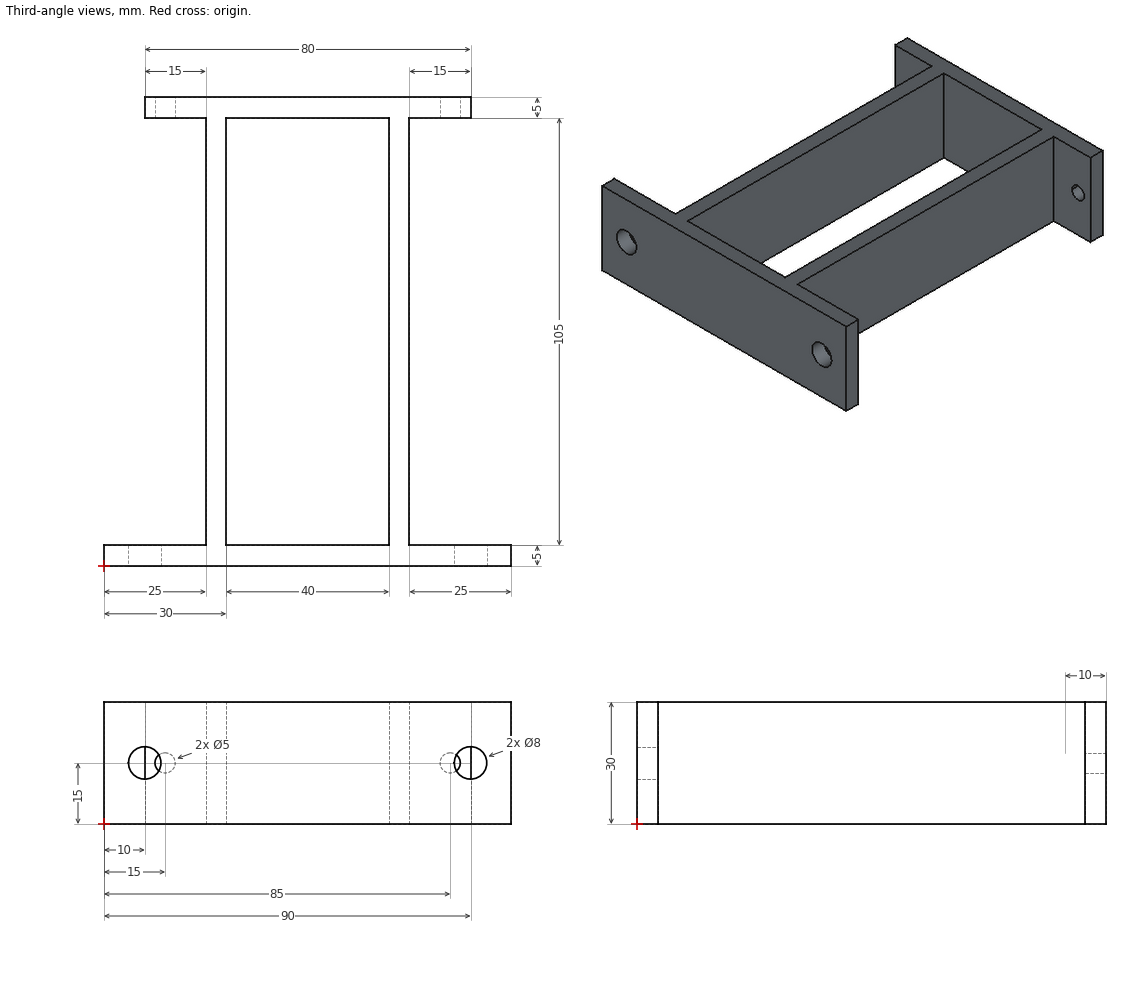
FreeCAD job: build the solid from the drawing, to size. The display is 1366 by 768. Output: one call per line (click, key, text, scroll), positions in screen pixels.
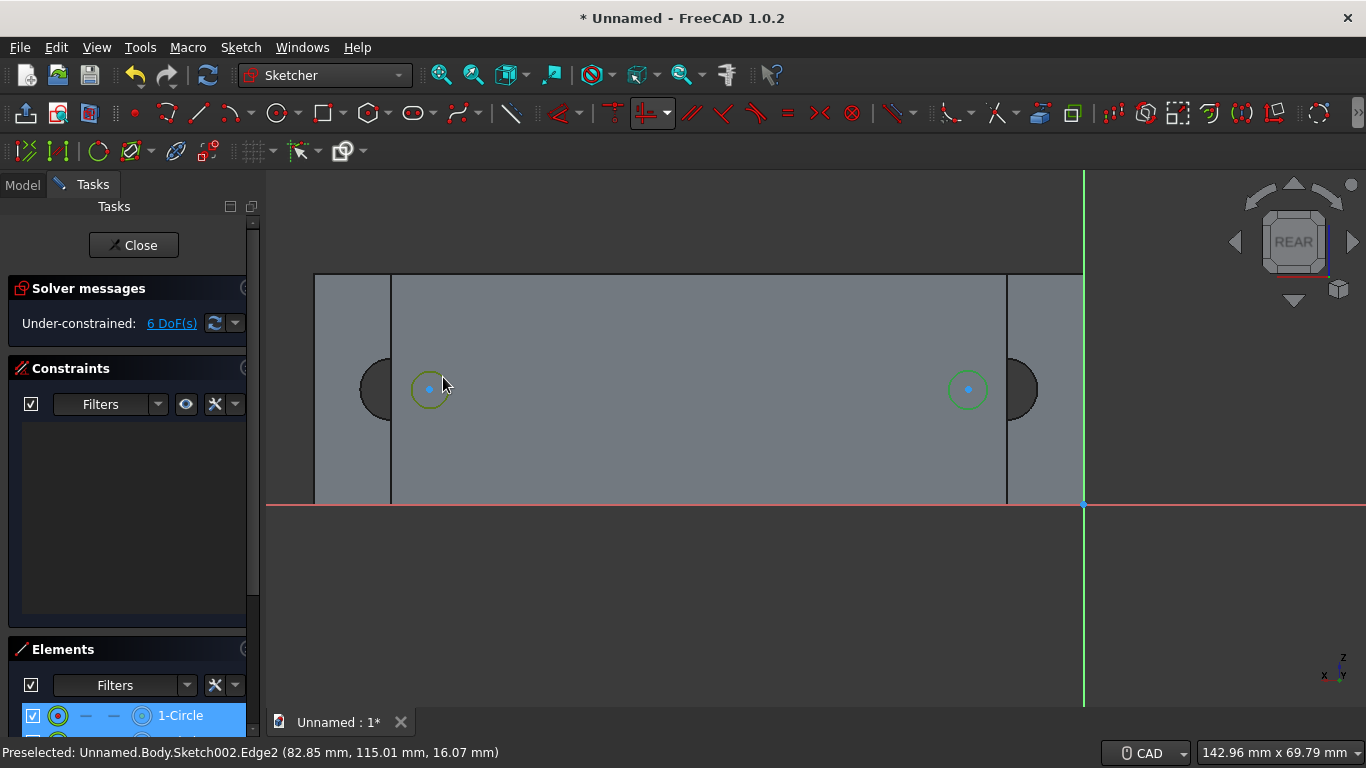
click(788, 114)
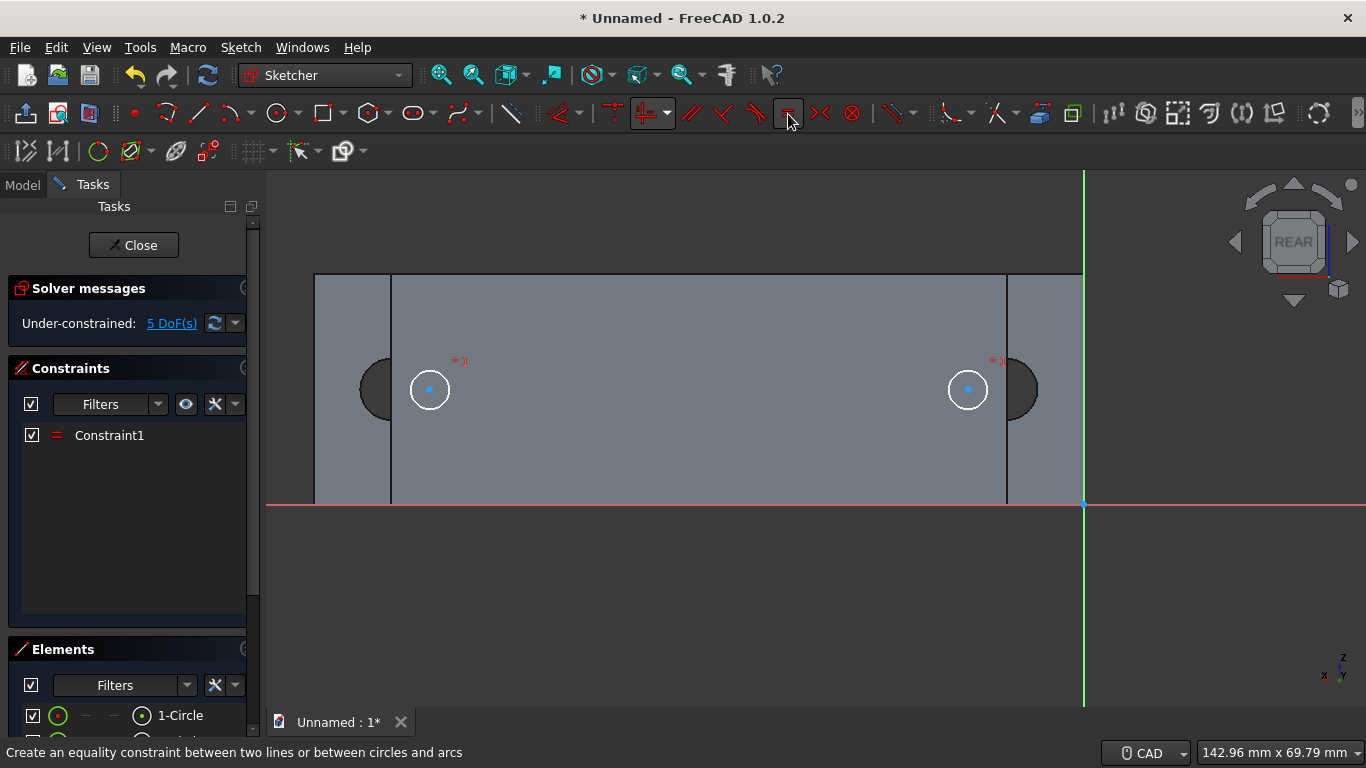
click(968, 390)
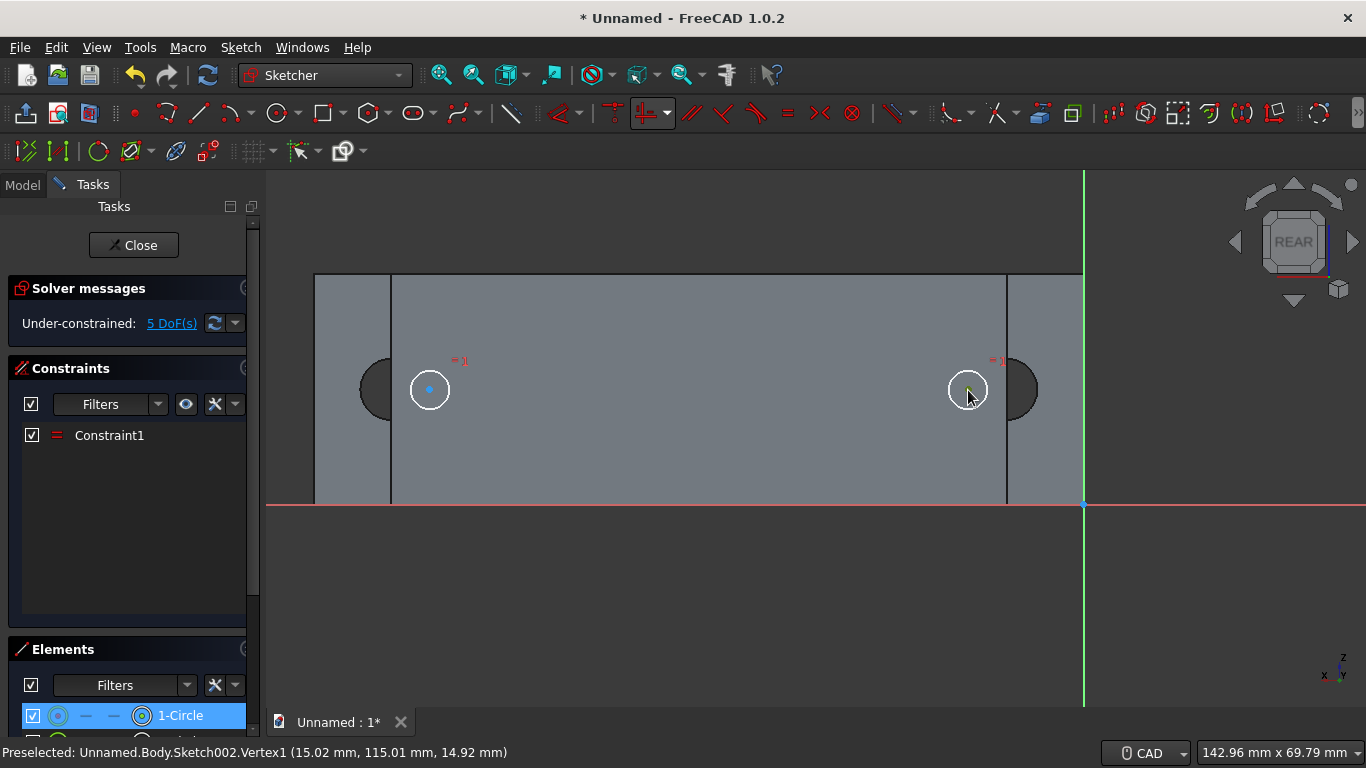
click(430, 390)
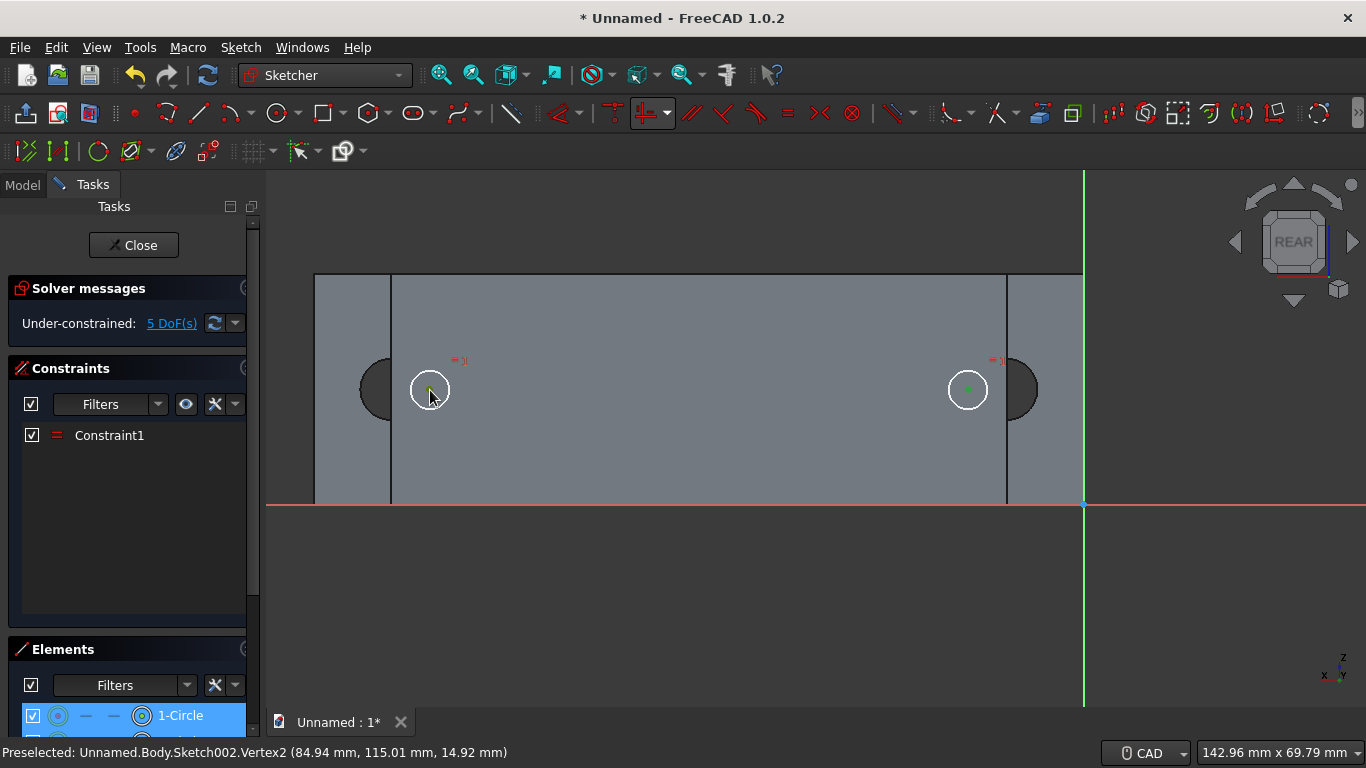
click(670, 114)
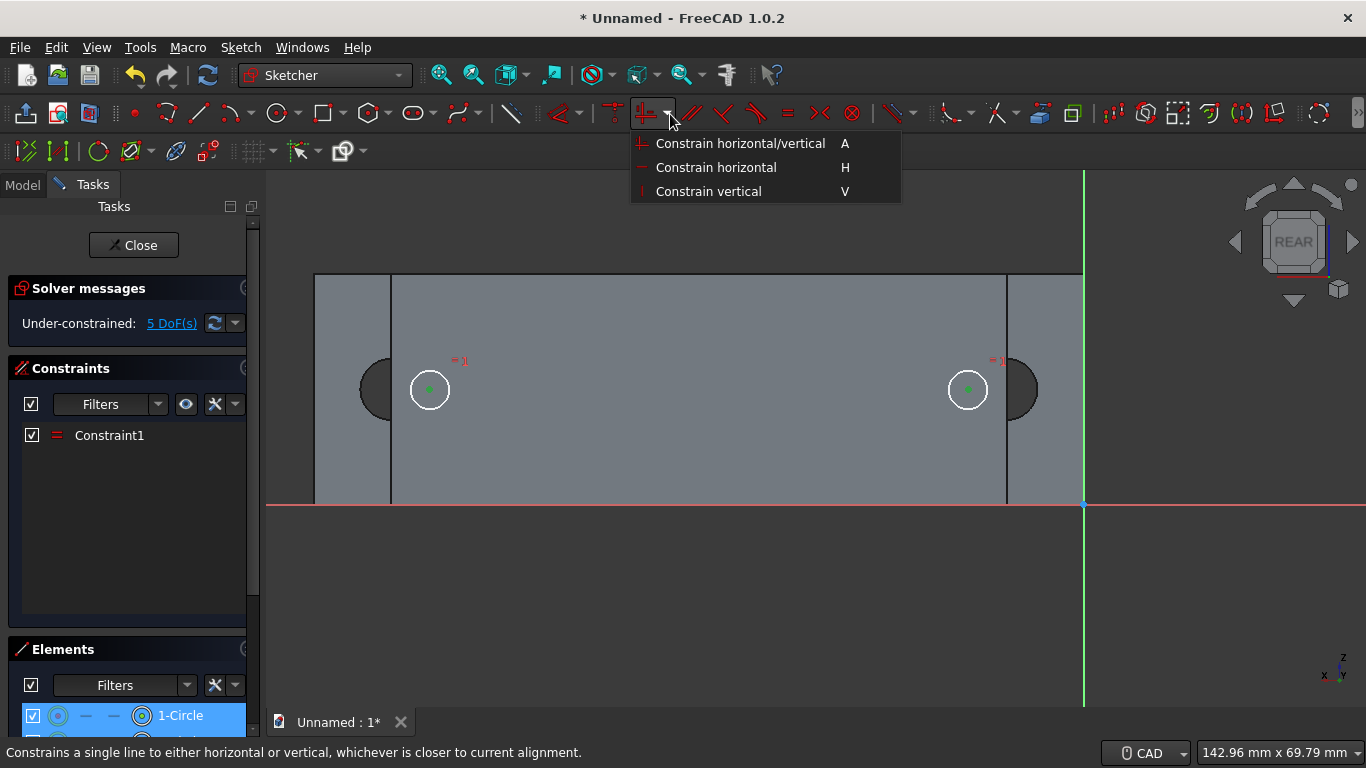
click(766, 167)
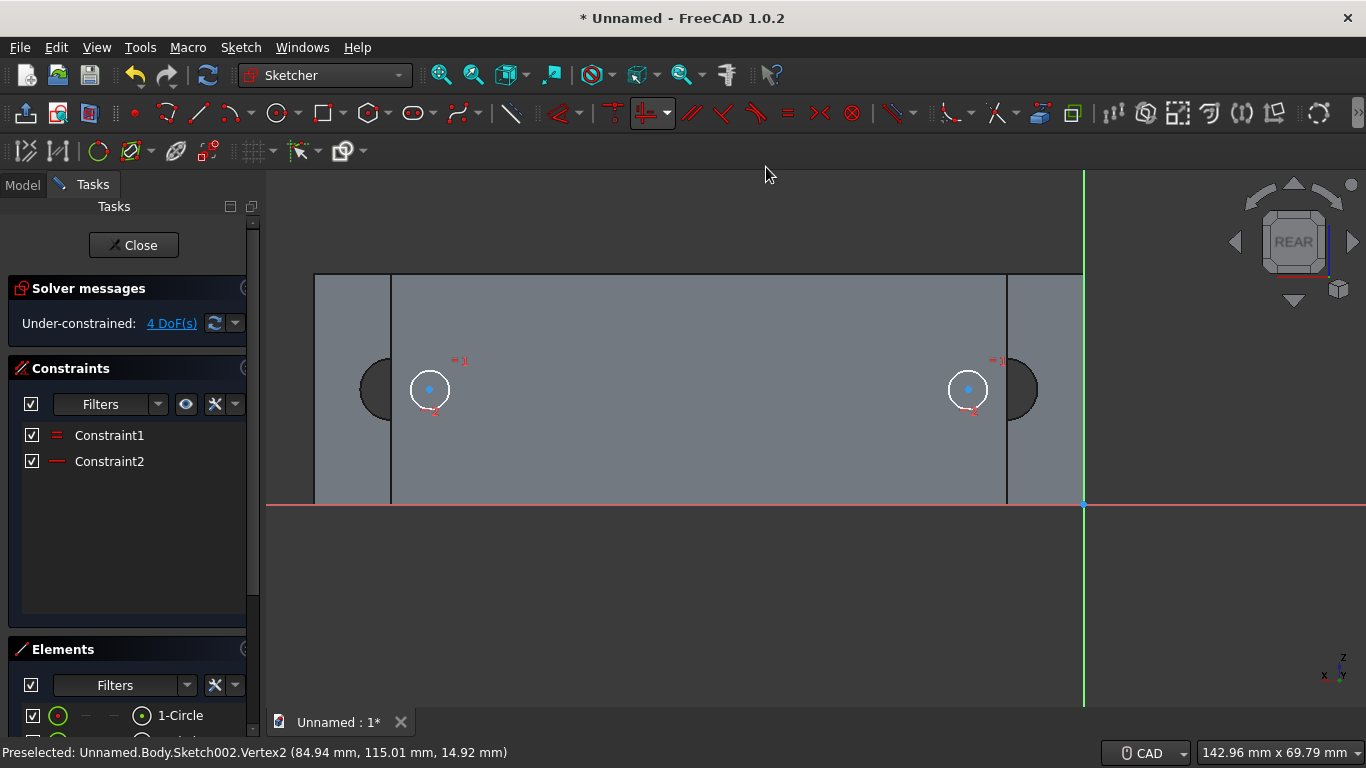
click(558, 114)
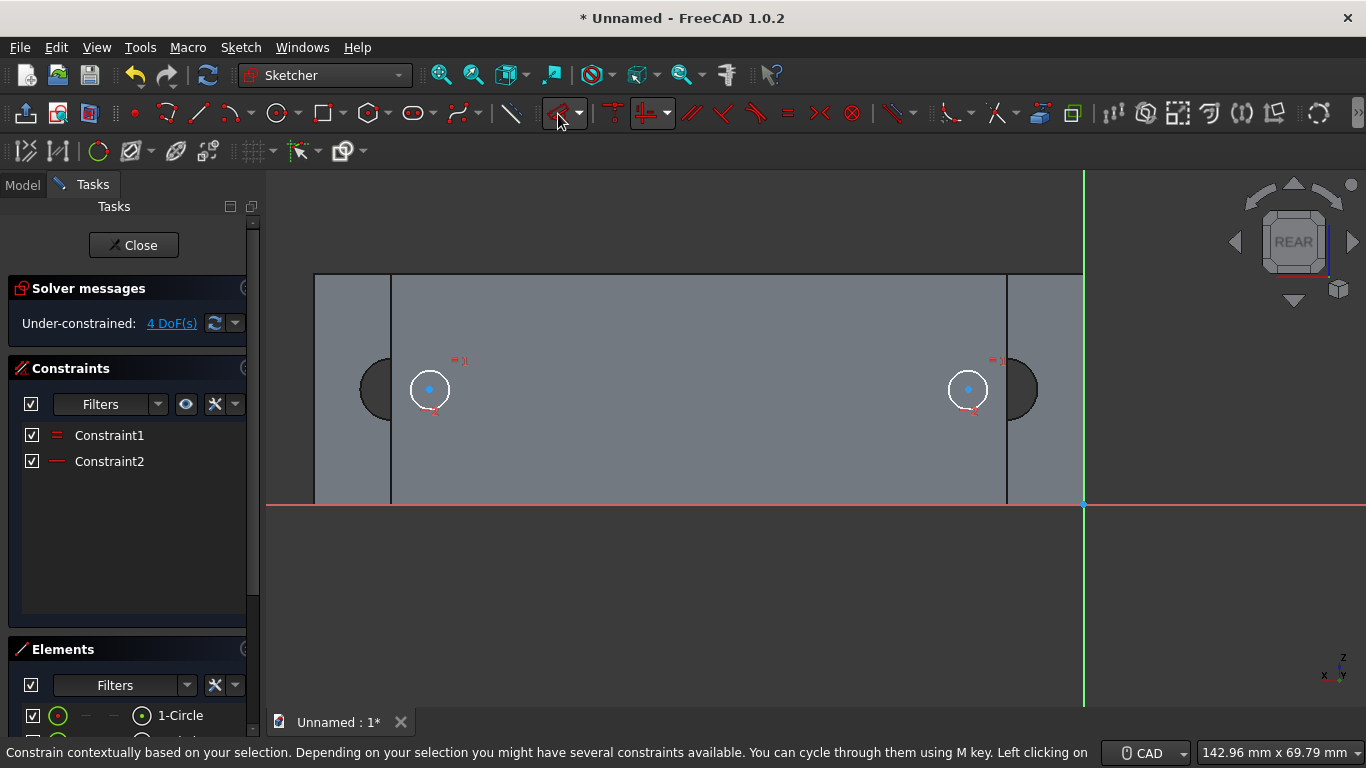
click(981, 376)
click(1003, 353)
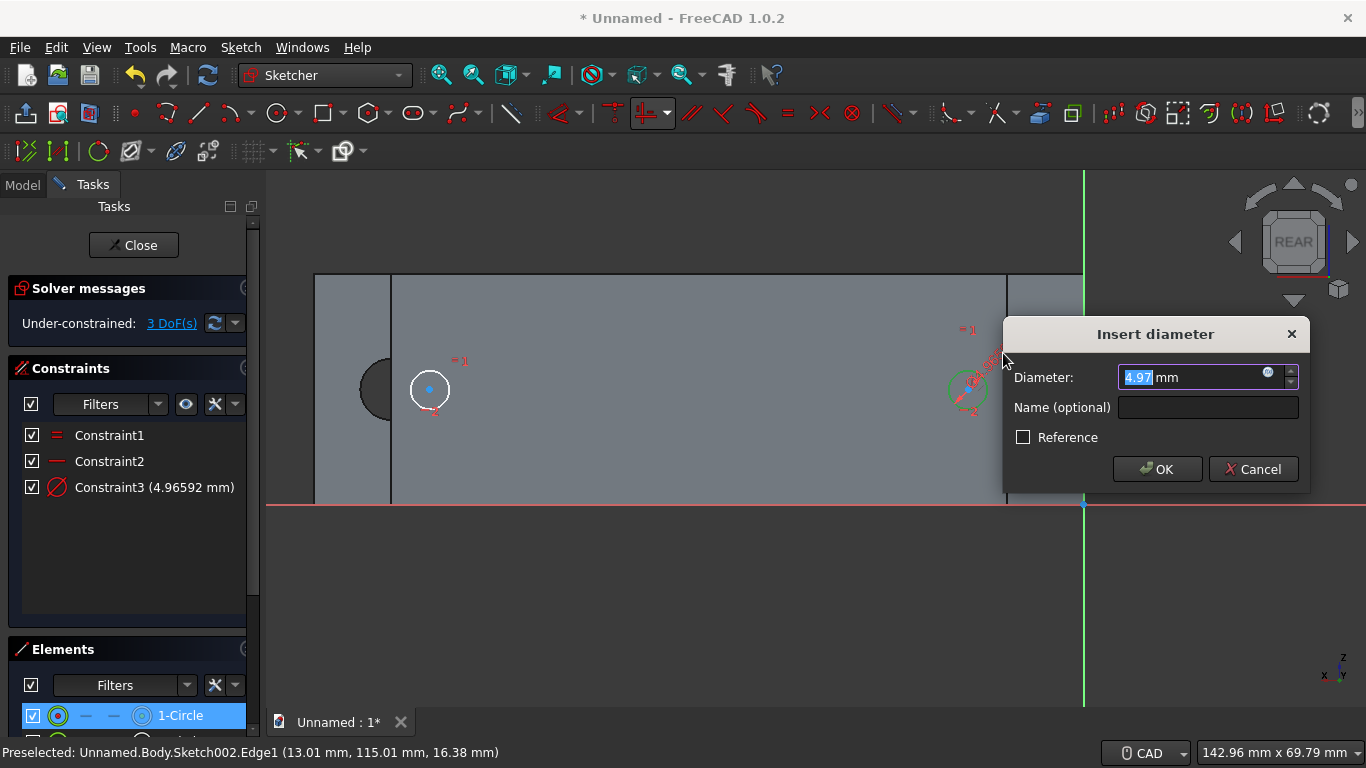
text(5)
key(Return)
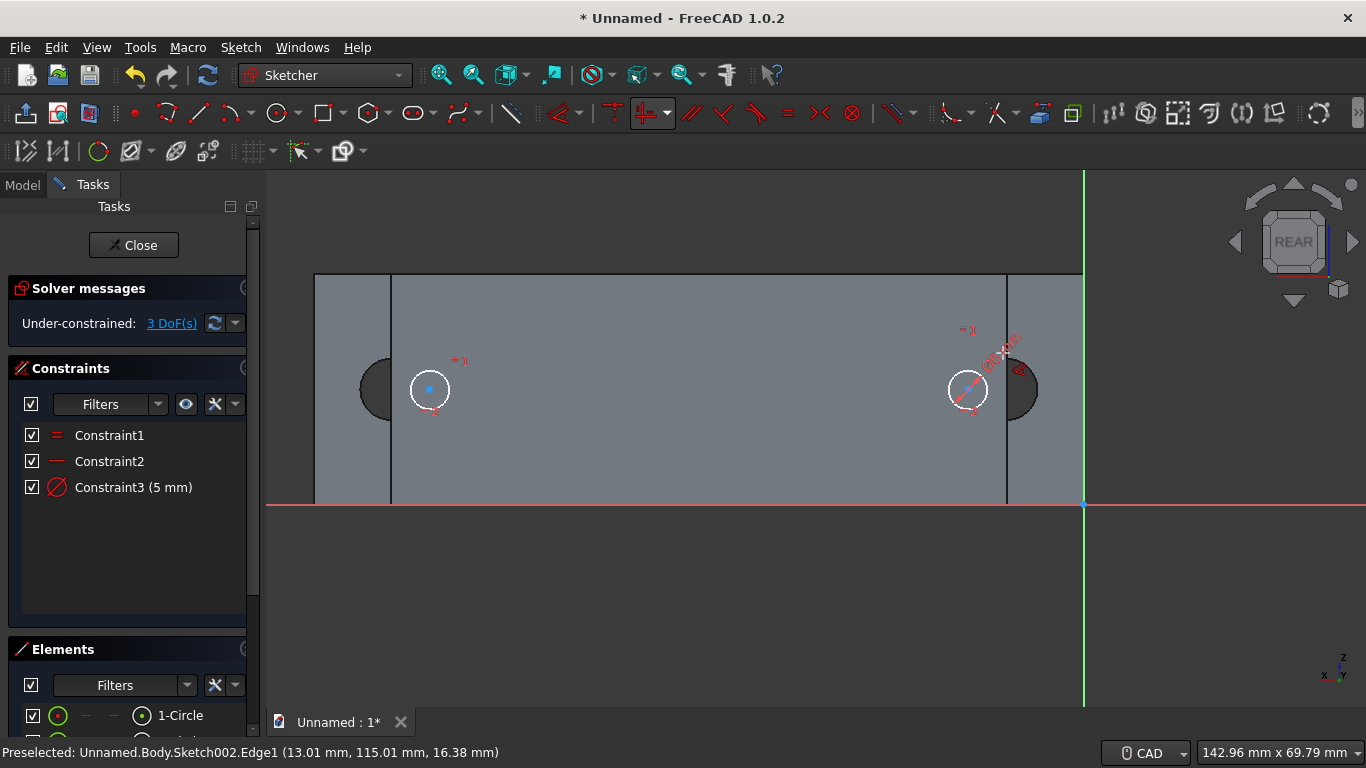
click(968, 390)
click(1026, 539)